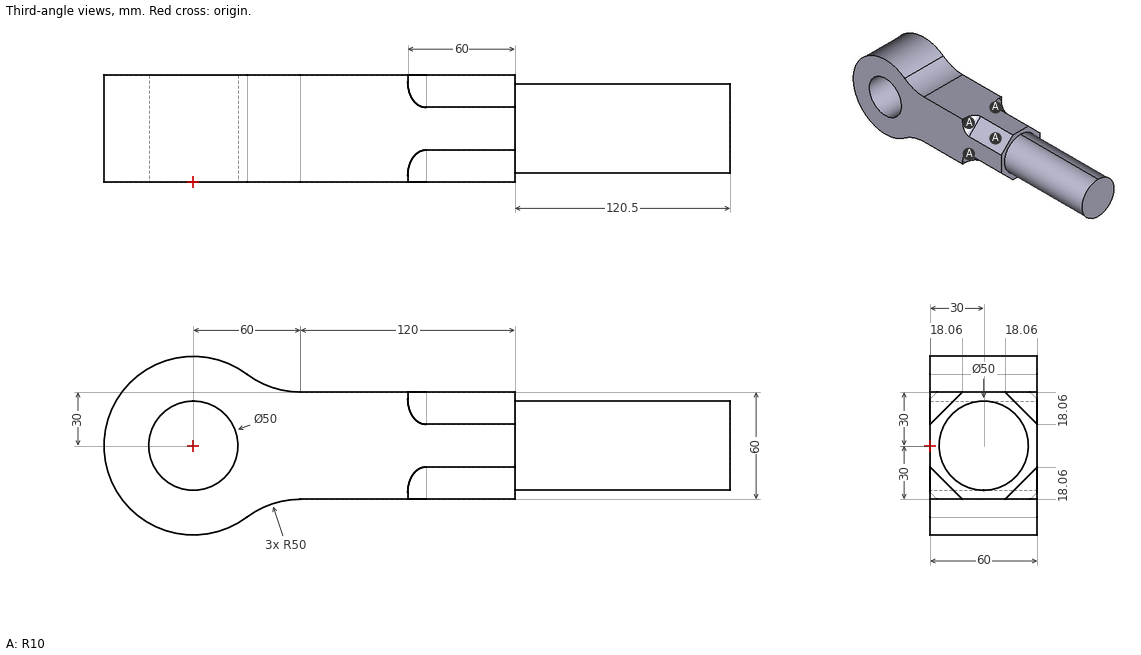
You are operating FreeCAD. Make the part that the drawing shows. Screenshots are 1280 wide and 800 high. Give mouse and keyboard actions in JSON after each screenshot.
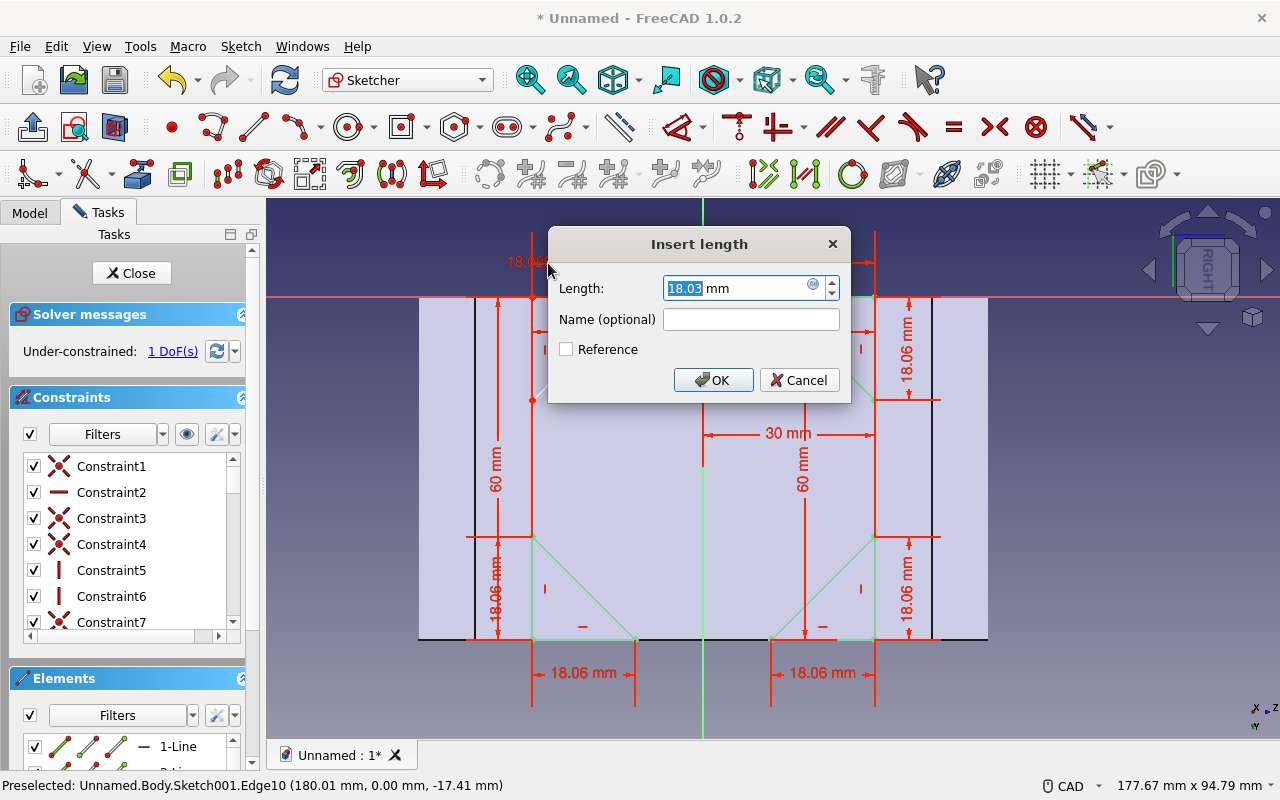
{"action": "type", "text": "18.06"}
{"action": "key", "text": "Return"}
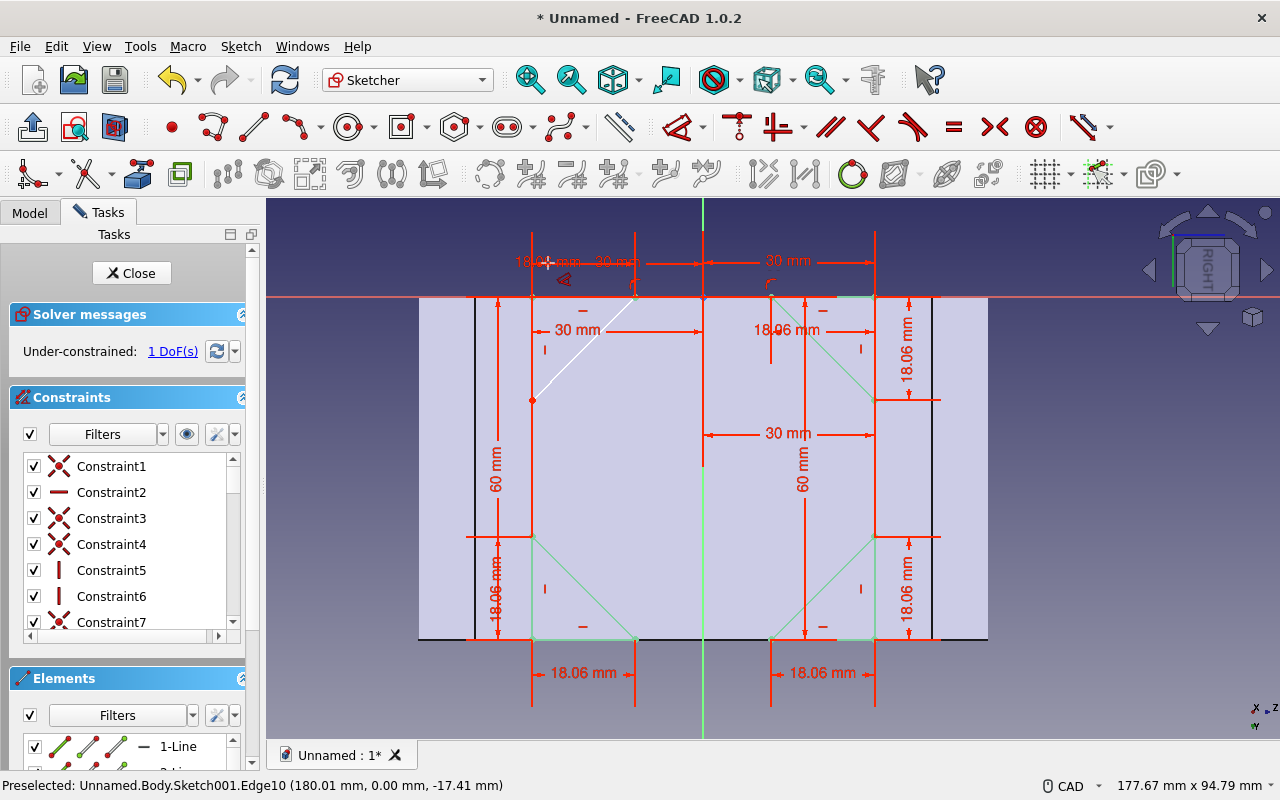
{"action": "left_click", "coordinate": [532, 328]}
{"action": "left_click", "coordinate": [498, 349]}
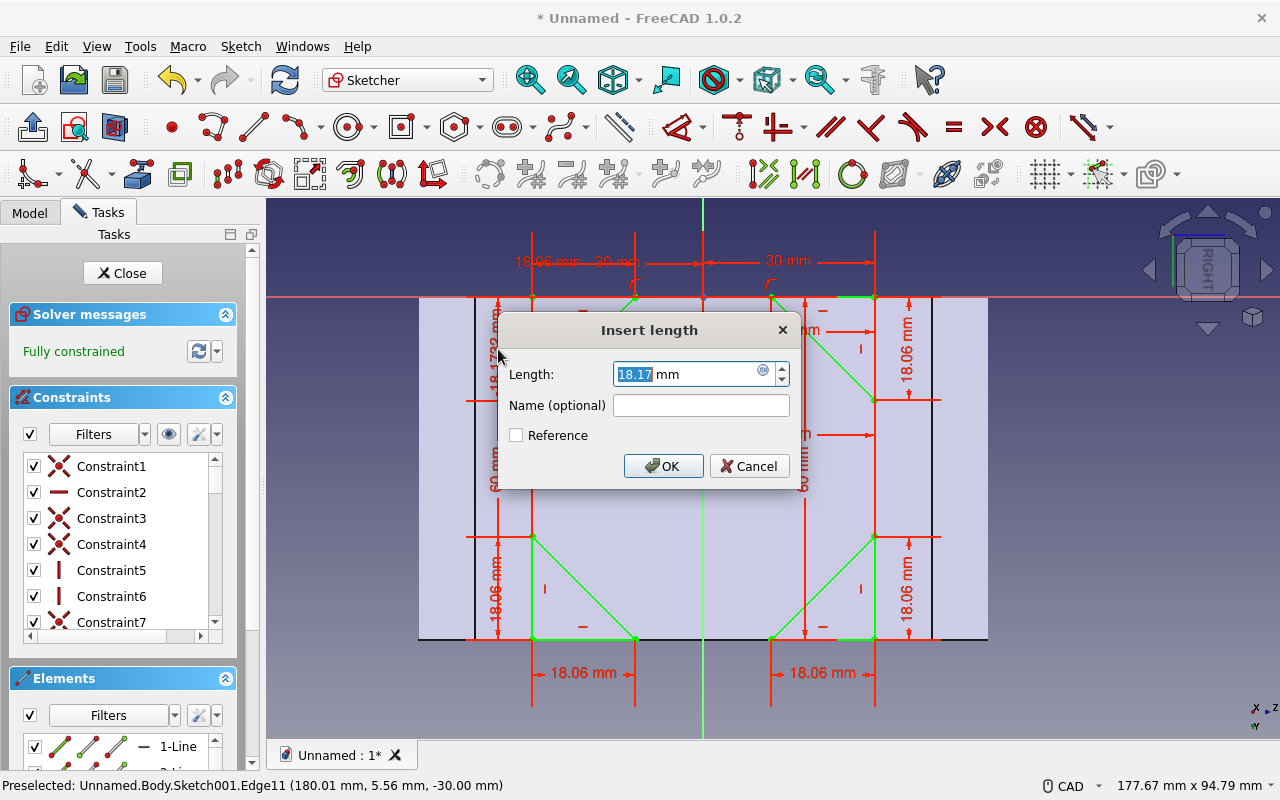
{"action": "type", "text": "18.06"}
{"action": "key", "text": "Return"}
{"action": "key", "text": "Escape"}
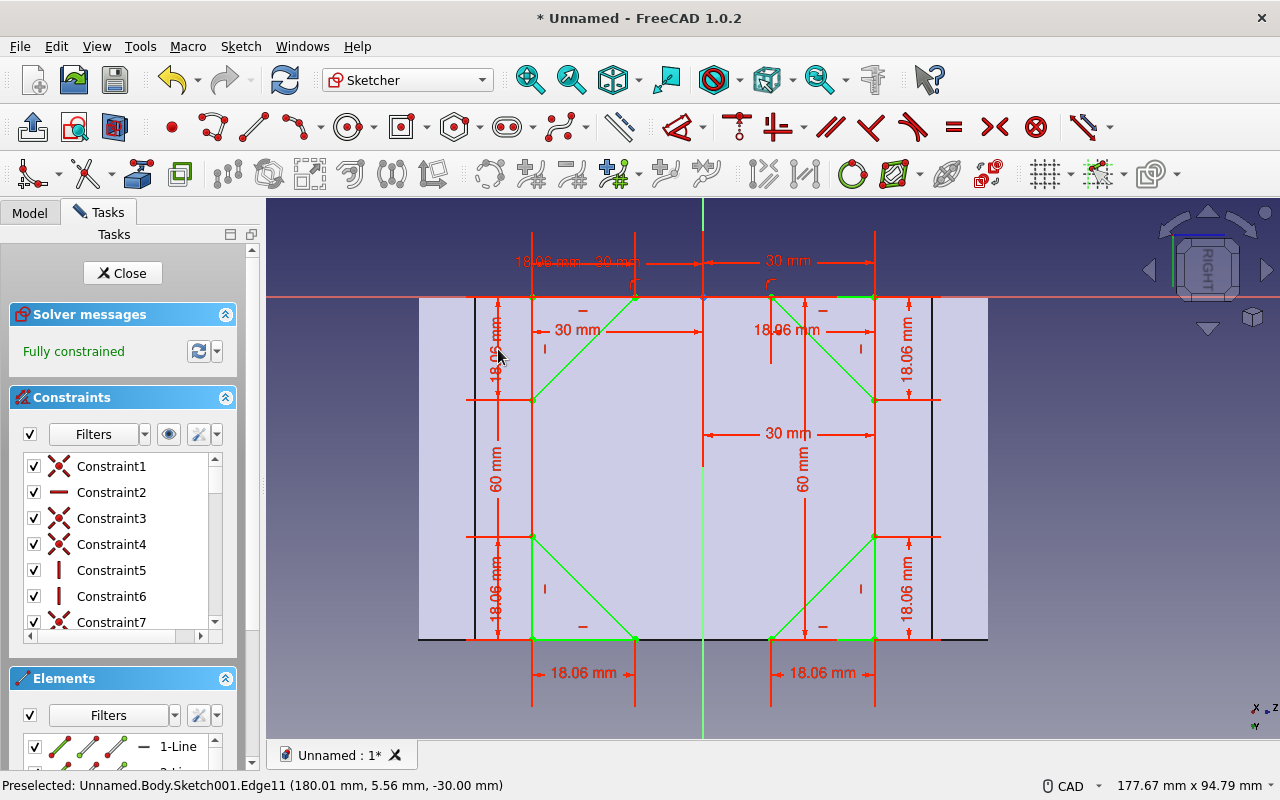
{"action": "left_click", "coordinate": [123, 273]}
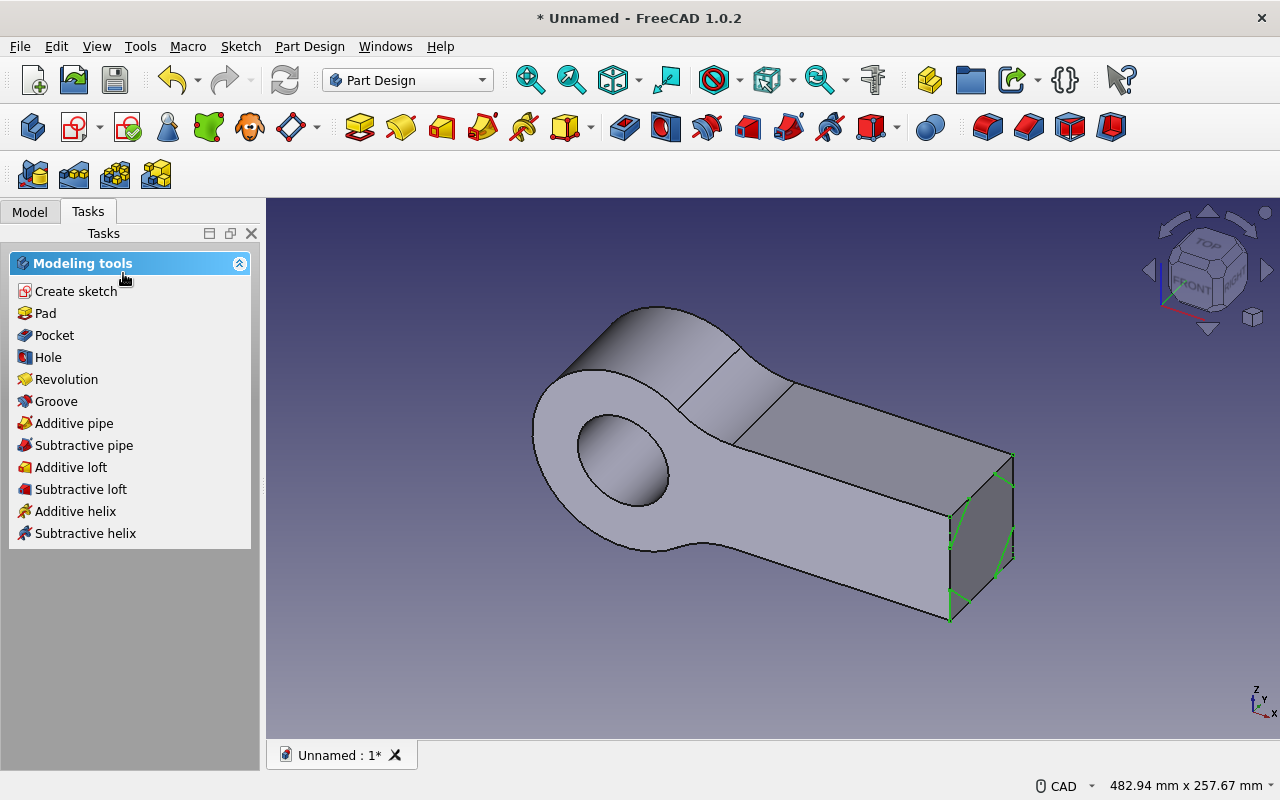
{"action": "left_click", "coordinate": [625, 128]}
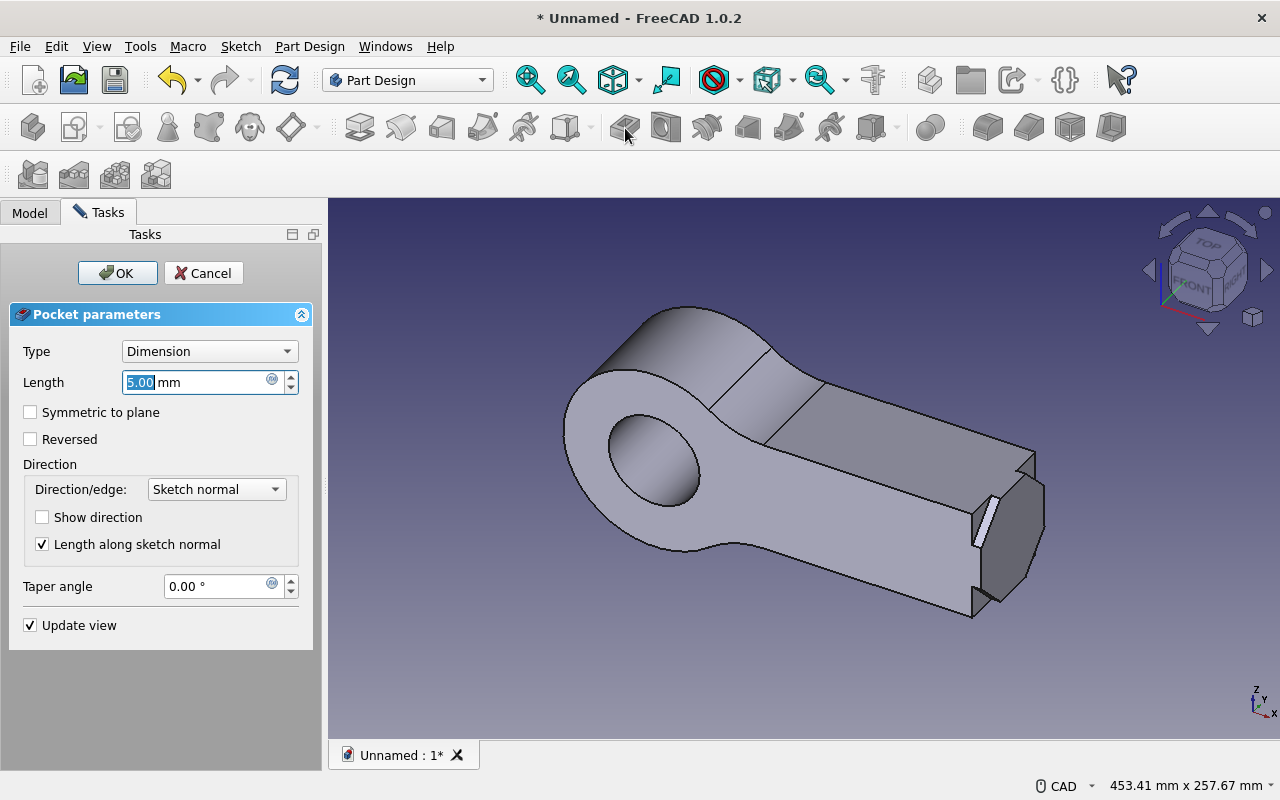
{"action": "type", "text": "60"}
{"action": "key", "text": "Tab"}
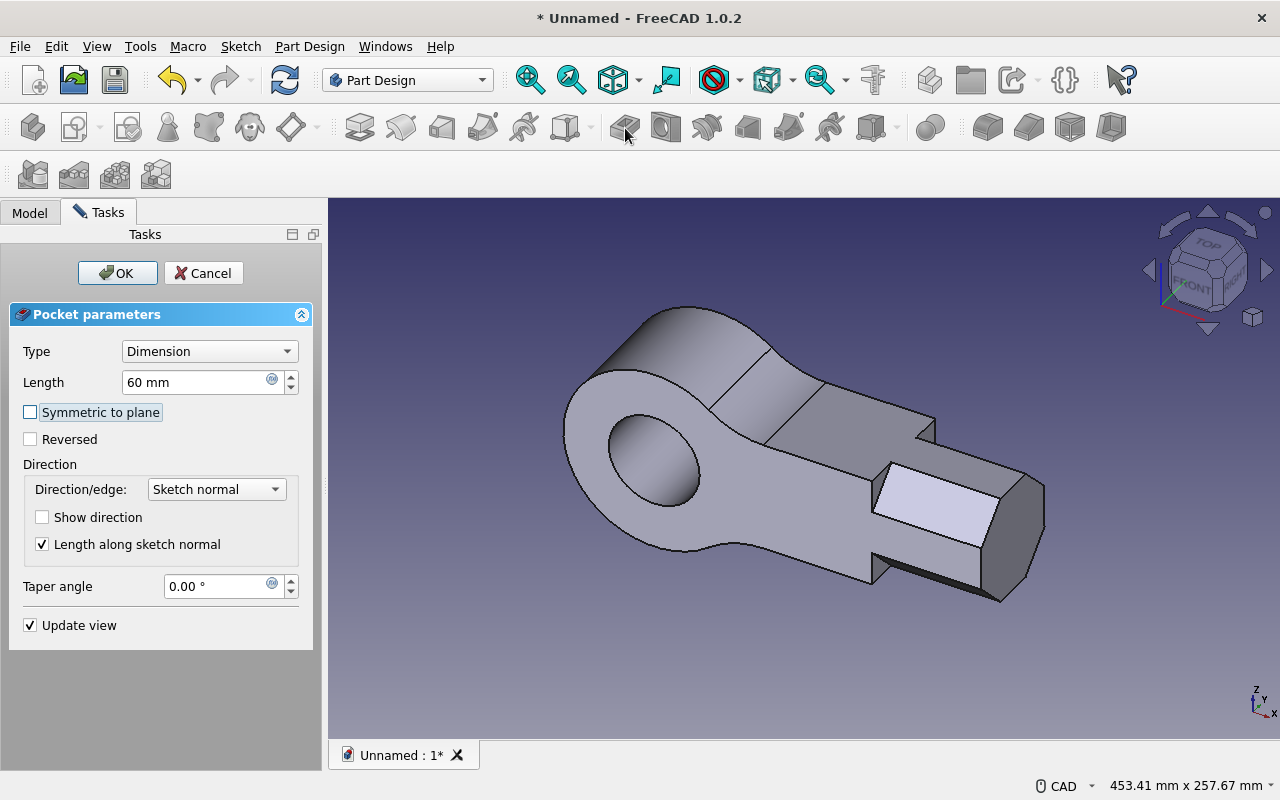
{"action": "left_click", "coordinate": [118, 273]}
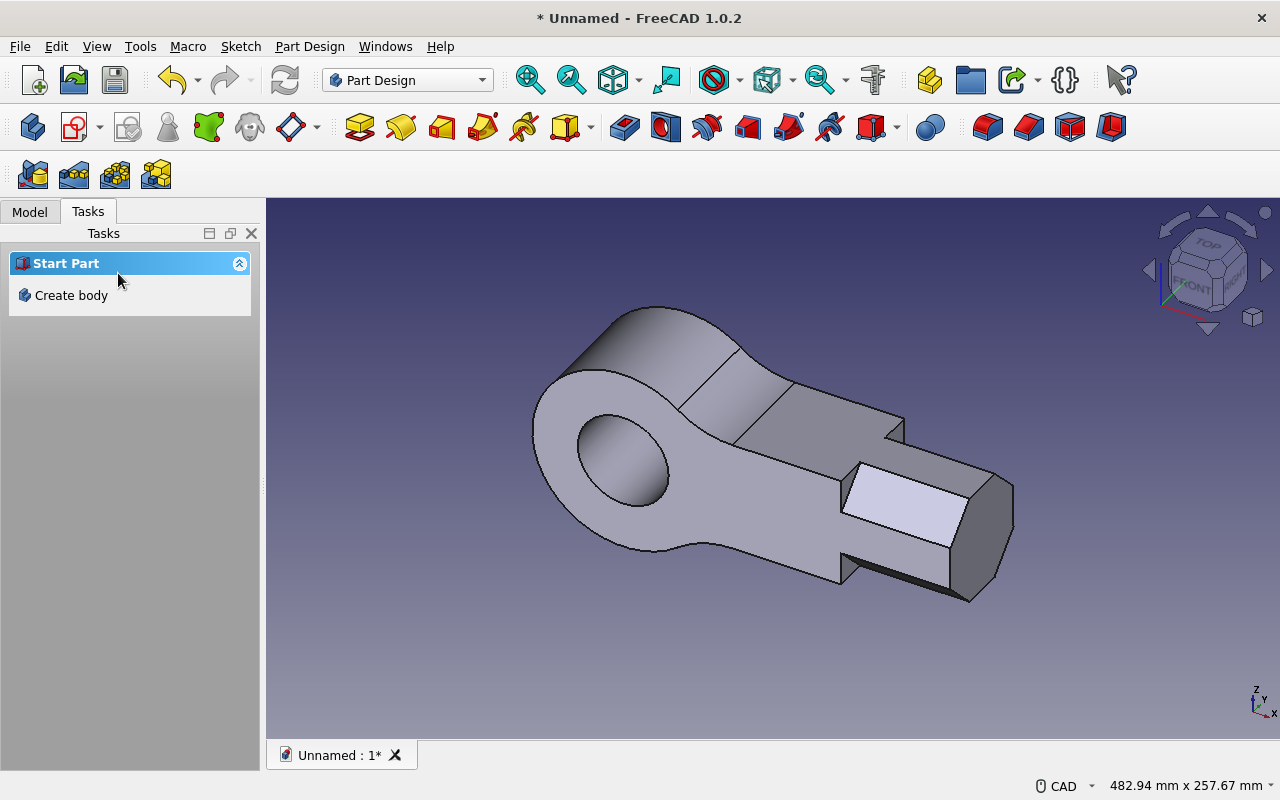
{"action": "left_click", "coordinate": [982, 537]}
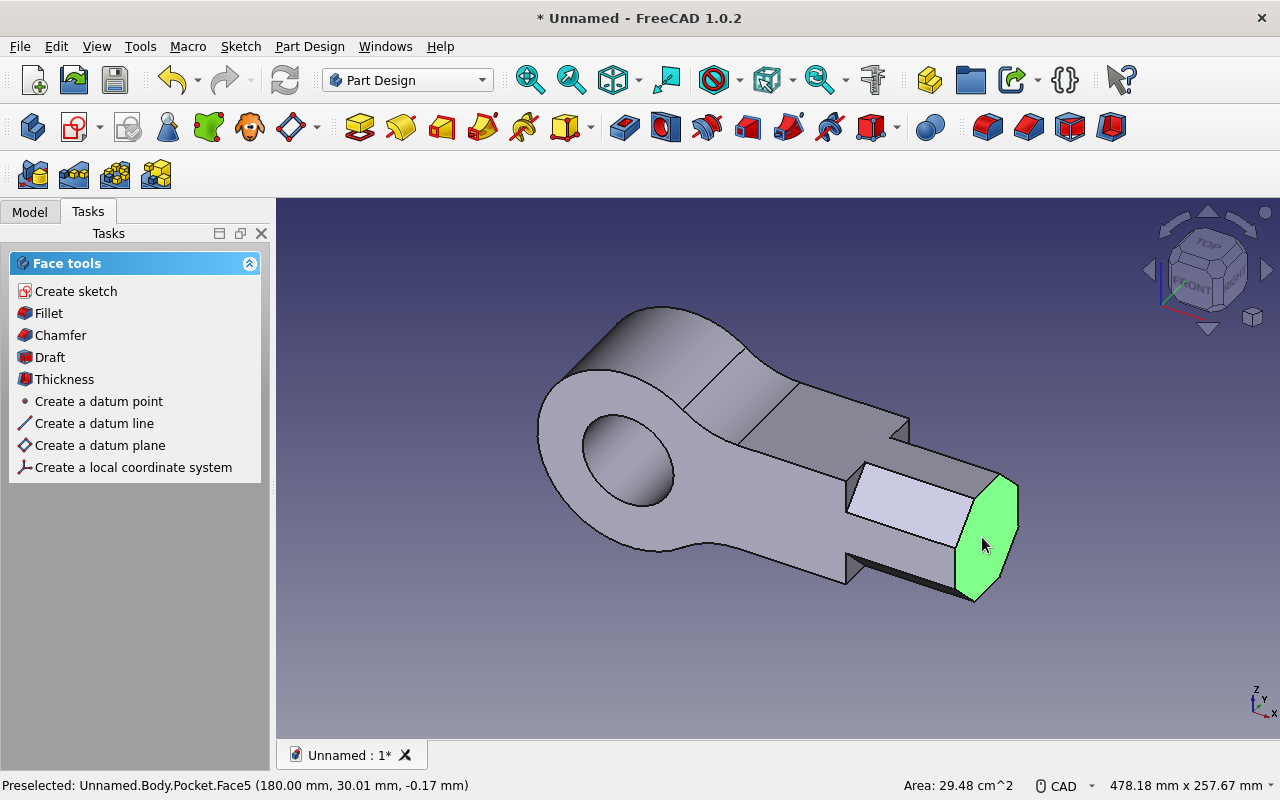
{"action": "left_click", "coordinate": [74, 128]}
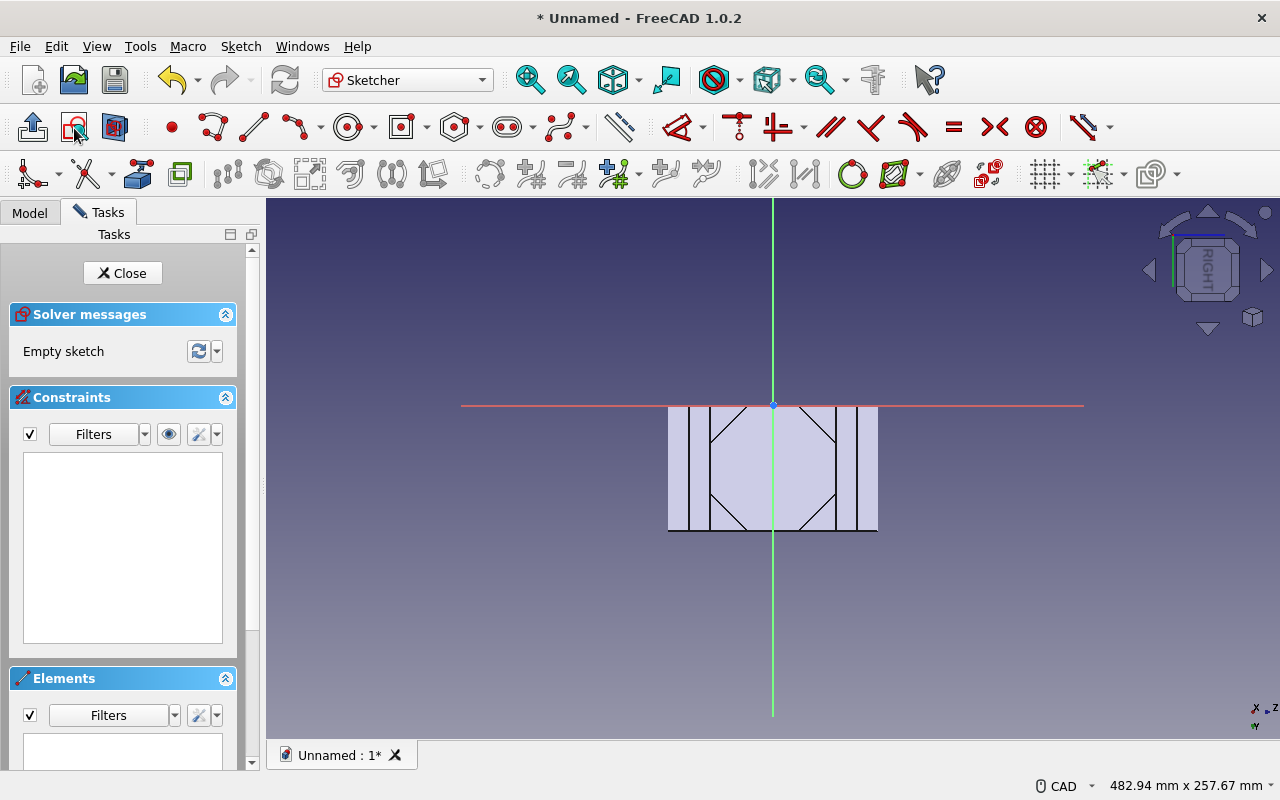
{"action": "scroll", "coordinate": [813, 460], "scroll_direction": "up", "scroll_amount": 5}